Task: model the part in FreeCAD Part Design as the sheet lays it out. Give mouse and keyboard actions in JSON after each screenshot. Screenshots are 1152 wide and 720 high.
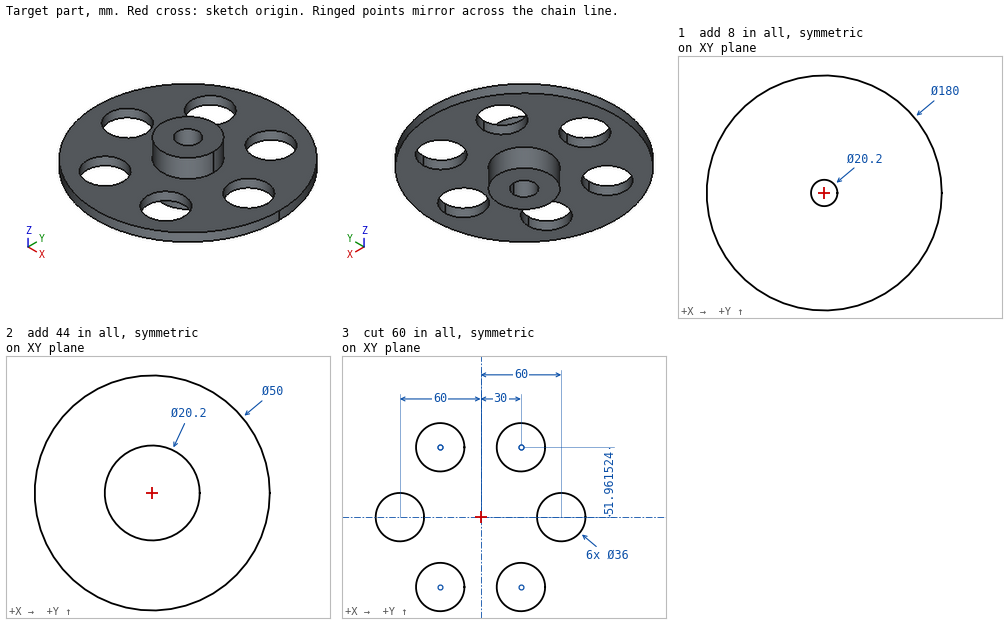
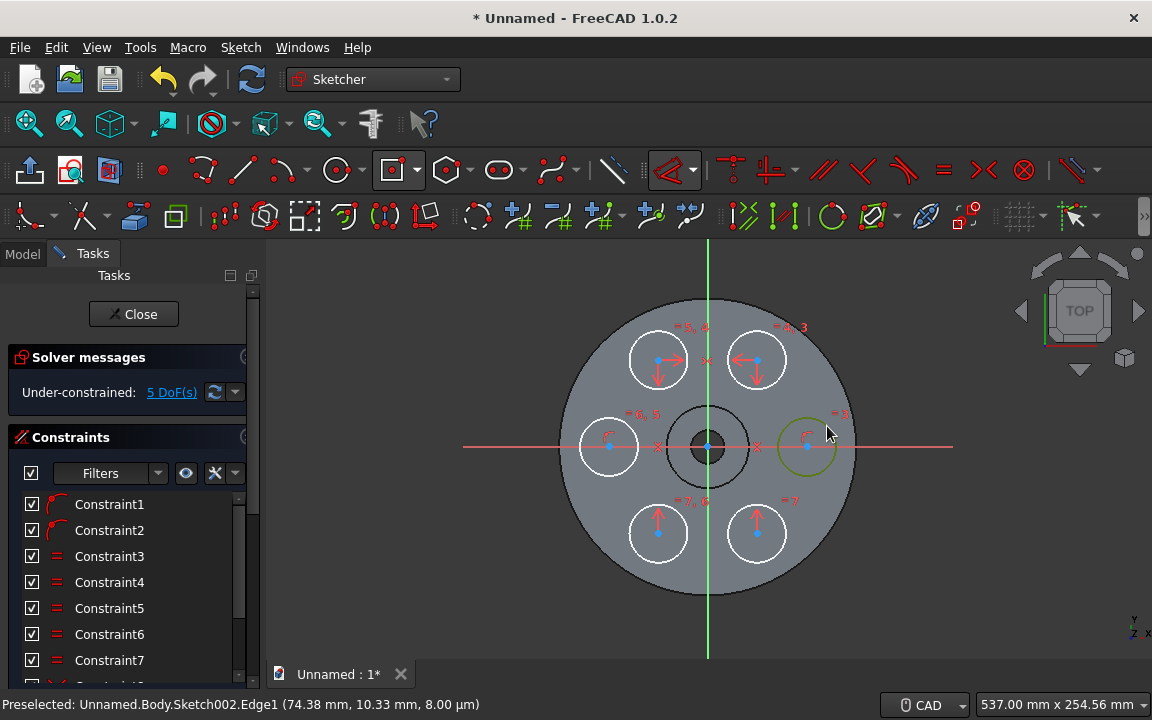
{"action": "key", "text": "k o"}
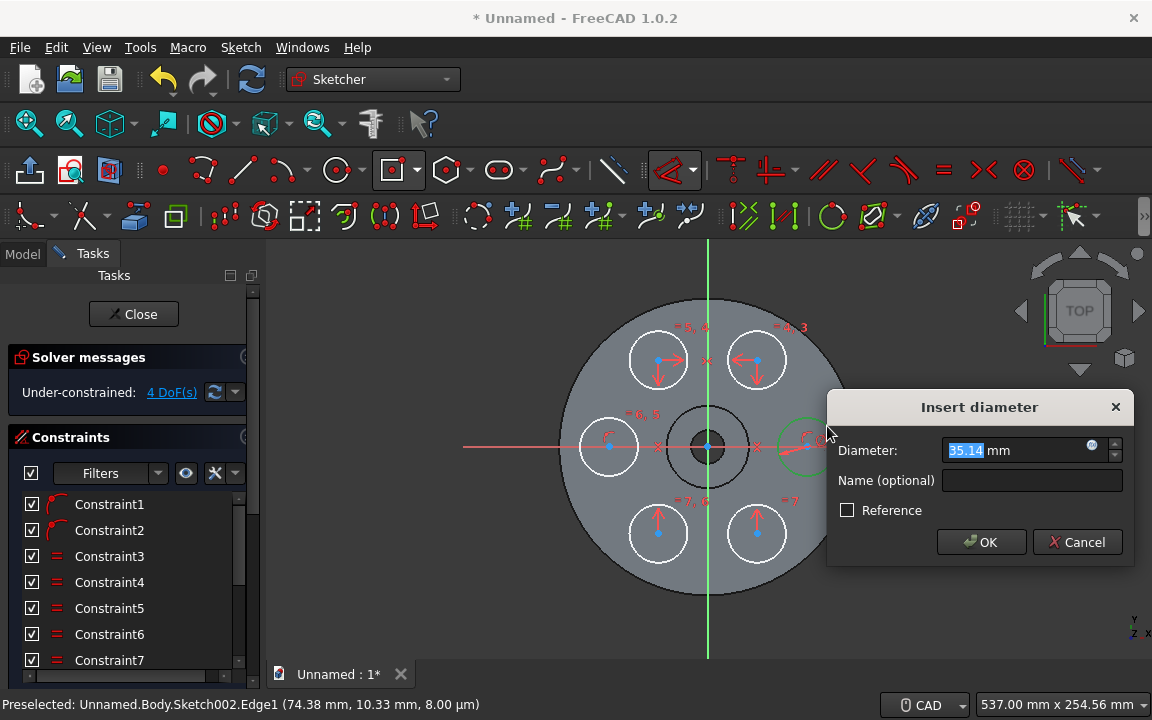
{"action": "type", "text": "36"}
{"action": "key", "text": "Return"}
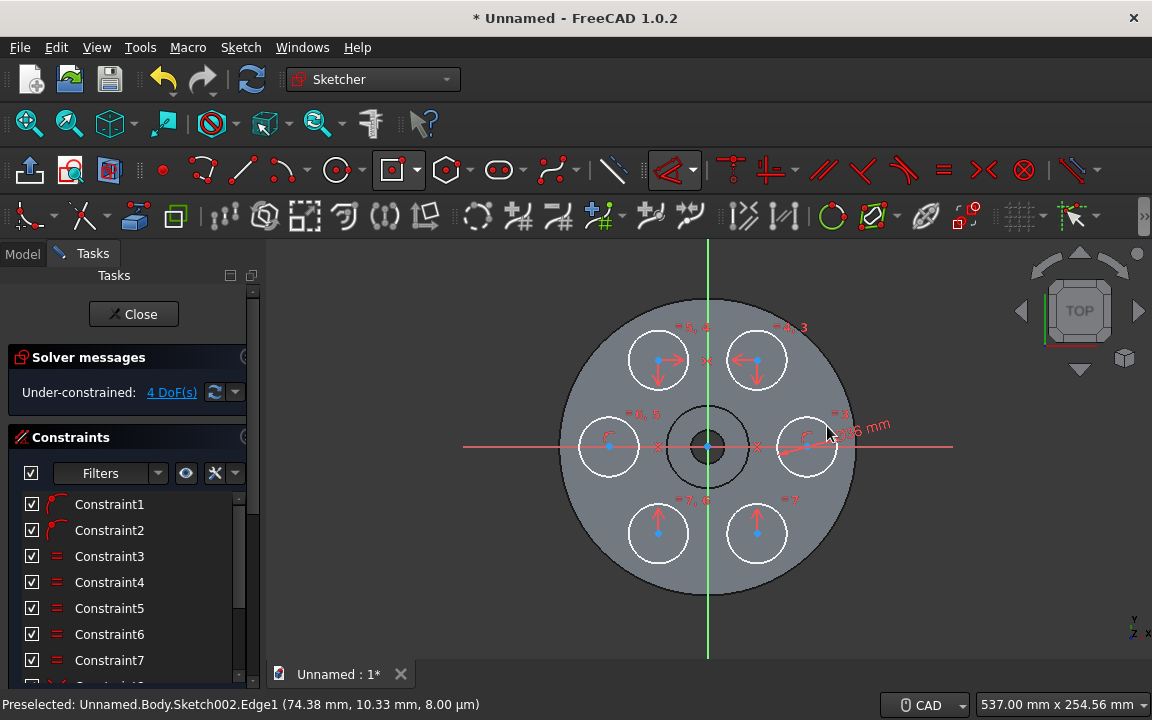
{"action": "left_click", "coordinate": [807, 447]}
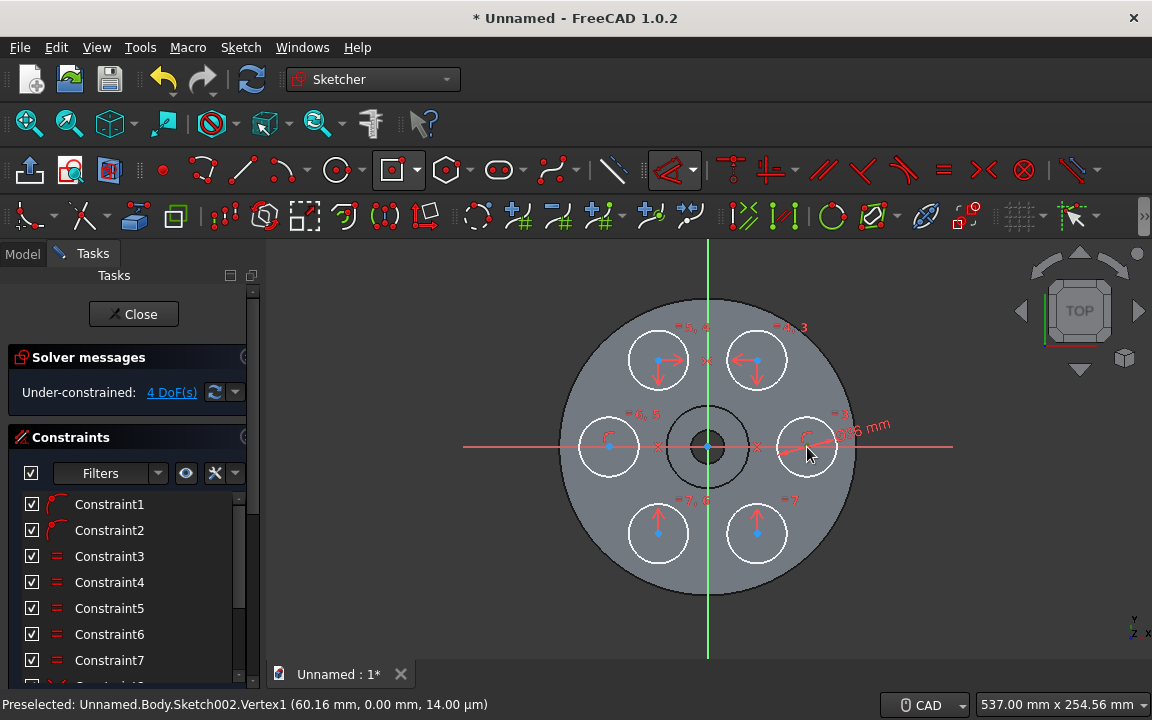
{"action": "key", "text": "l"}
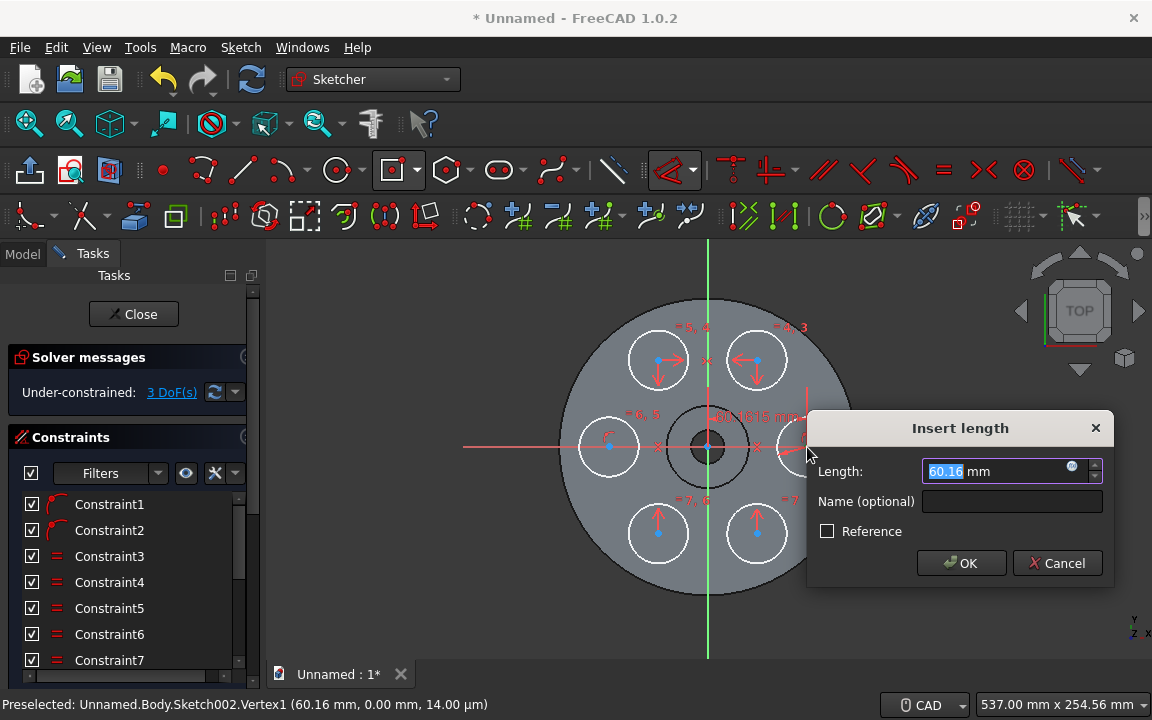
{"action": "type", "text": "60"}
{"action": "key", "text": "Return"}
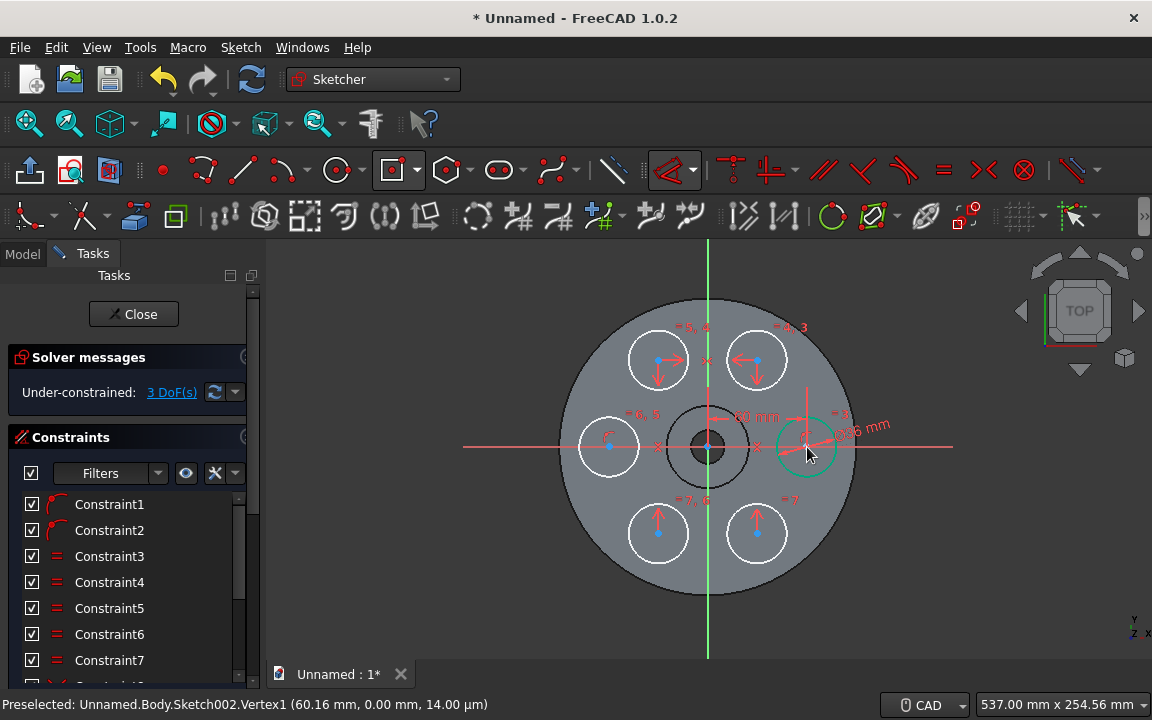
{"action": "left_click", "coordinate": [757, 360]}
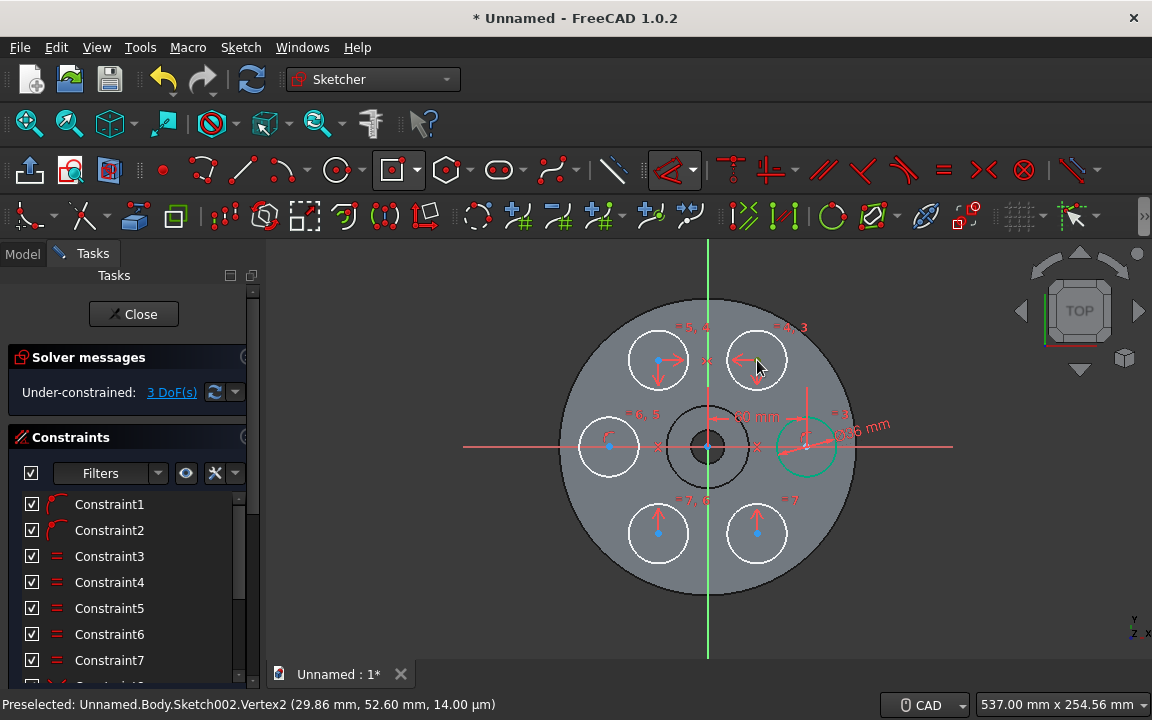
{"action": "key", "text": "l"}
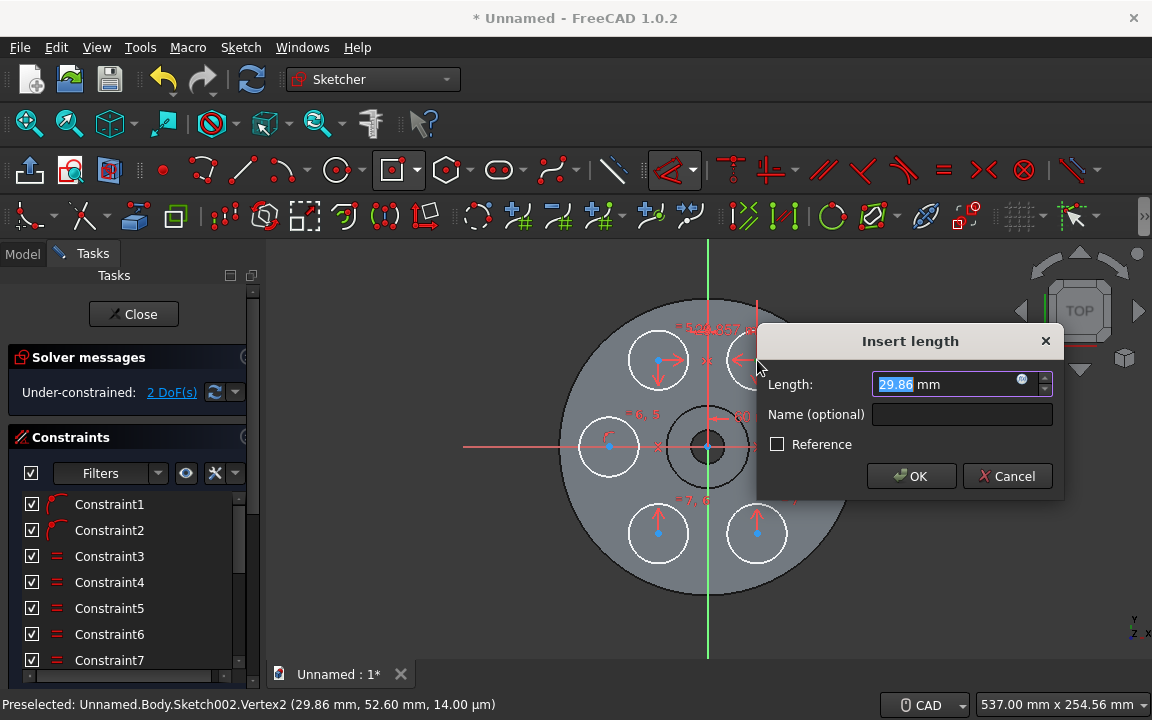
{"action": "type", "text": "30"}
{"action": "key", "text": "Return"}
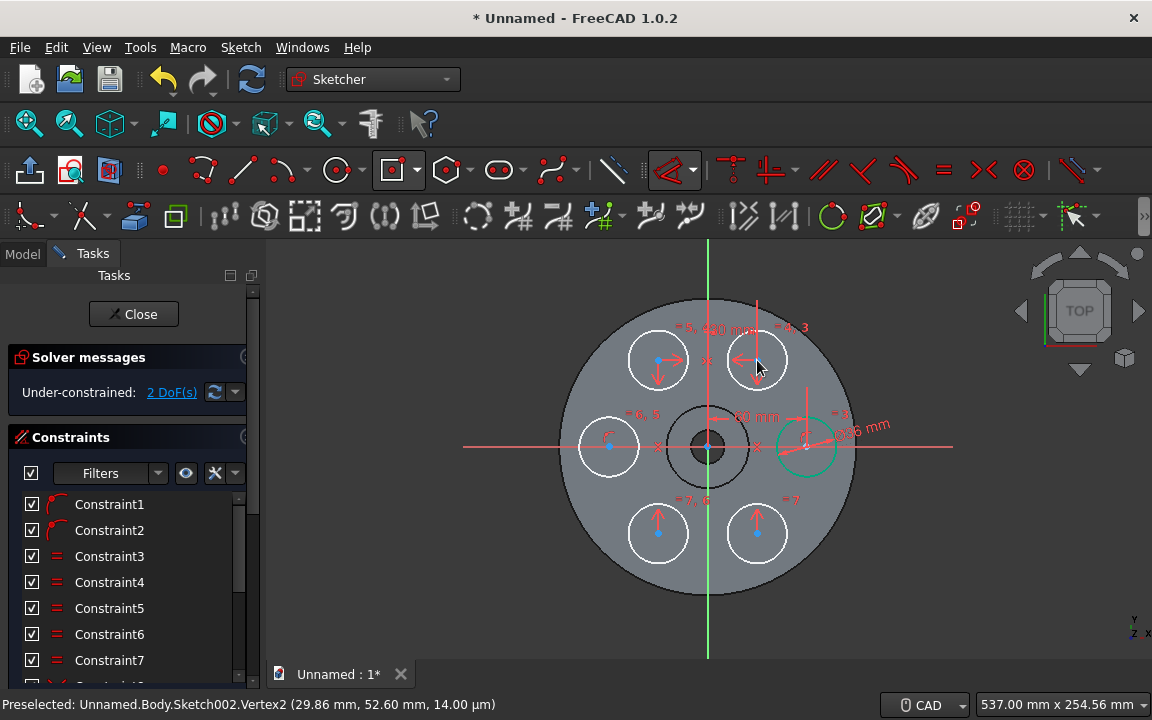
{"action": "left_click", "coordinate": [609, 447]}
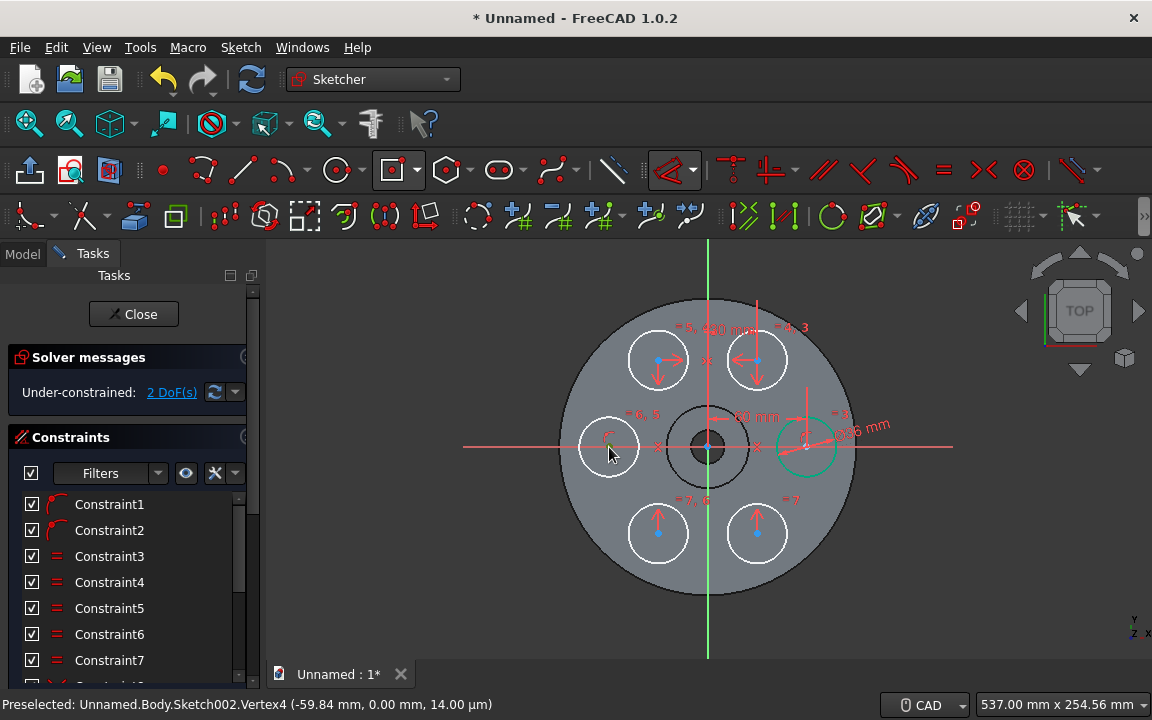
{"action": "left_click", "coordinate": [696, 170]}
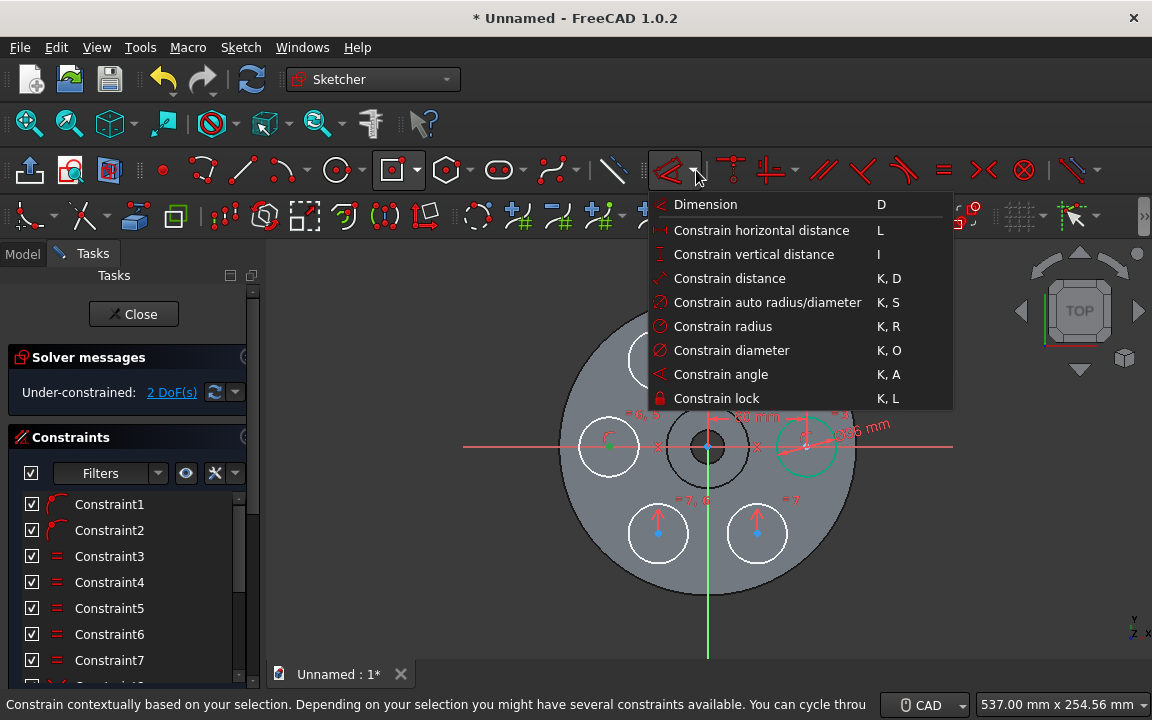
{"action": "left_click", "coordinate": [801, 230]}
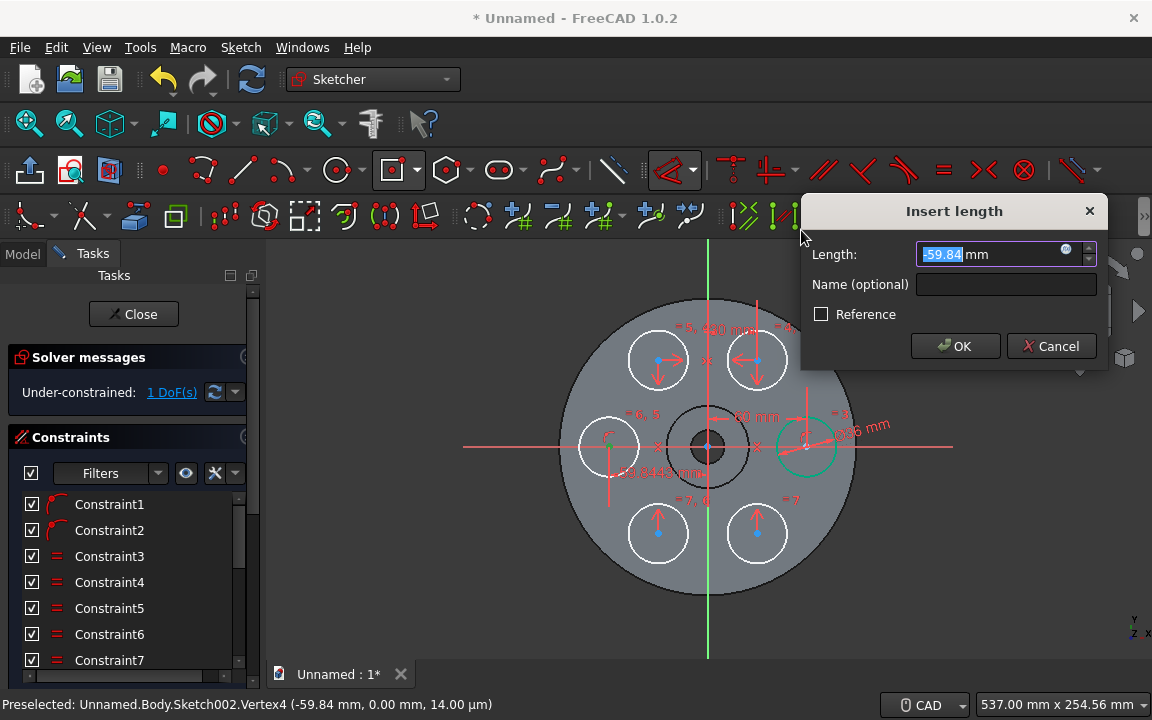
{"action": "type", "text": "-60"}
{"action": "key", "text": "Return"}